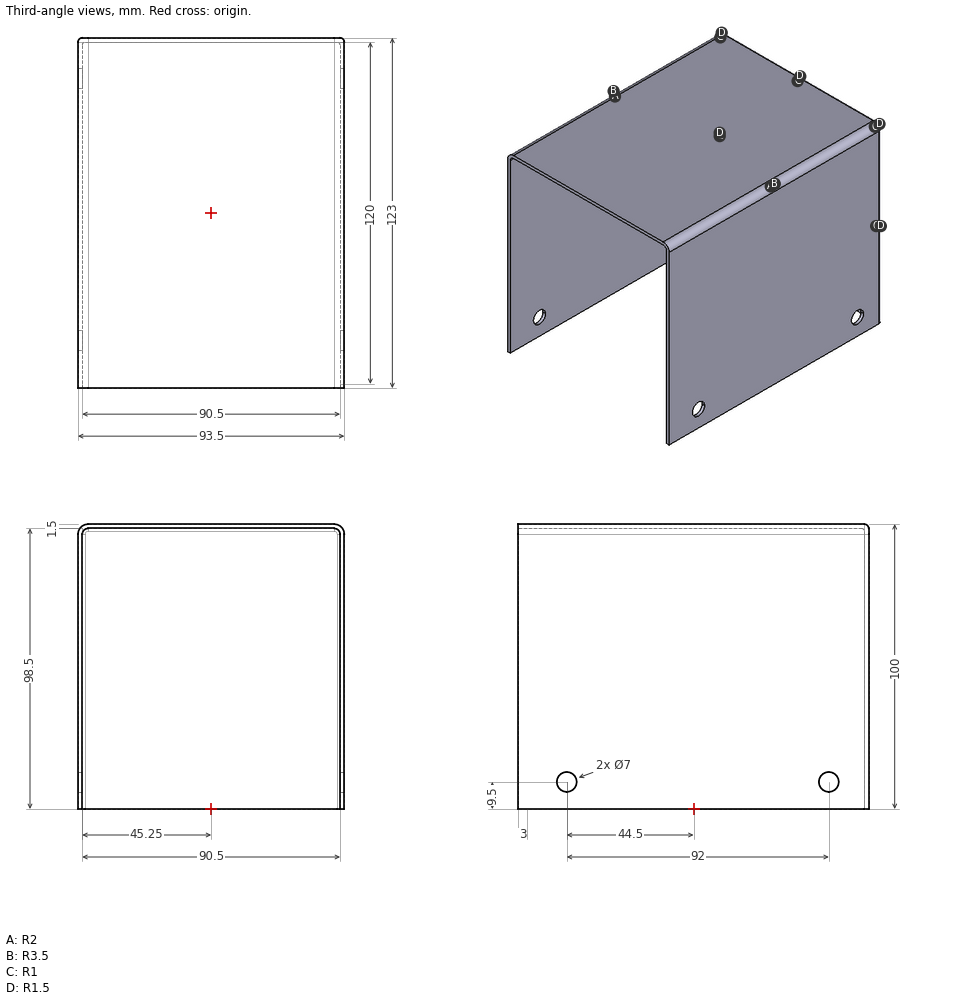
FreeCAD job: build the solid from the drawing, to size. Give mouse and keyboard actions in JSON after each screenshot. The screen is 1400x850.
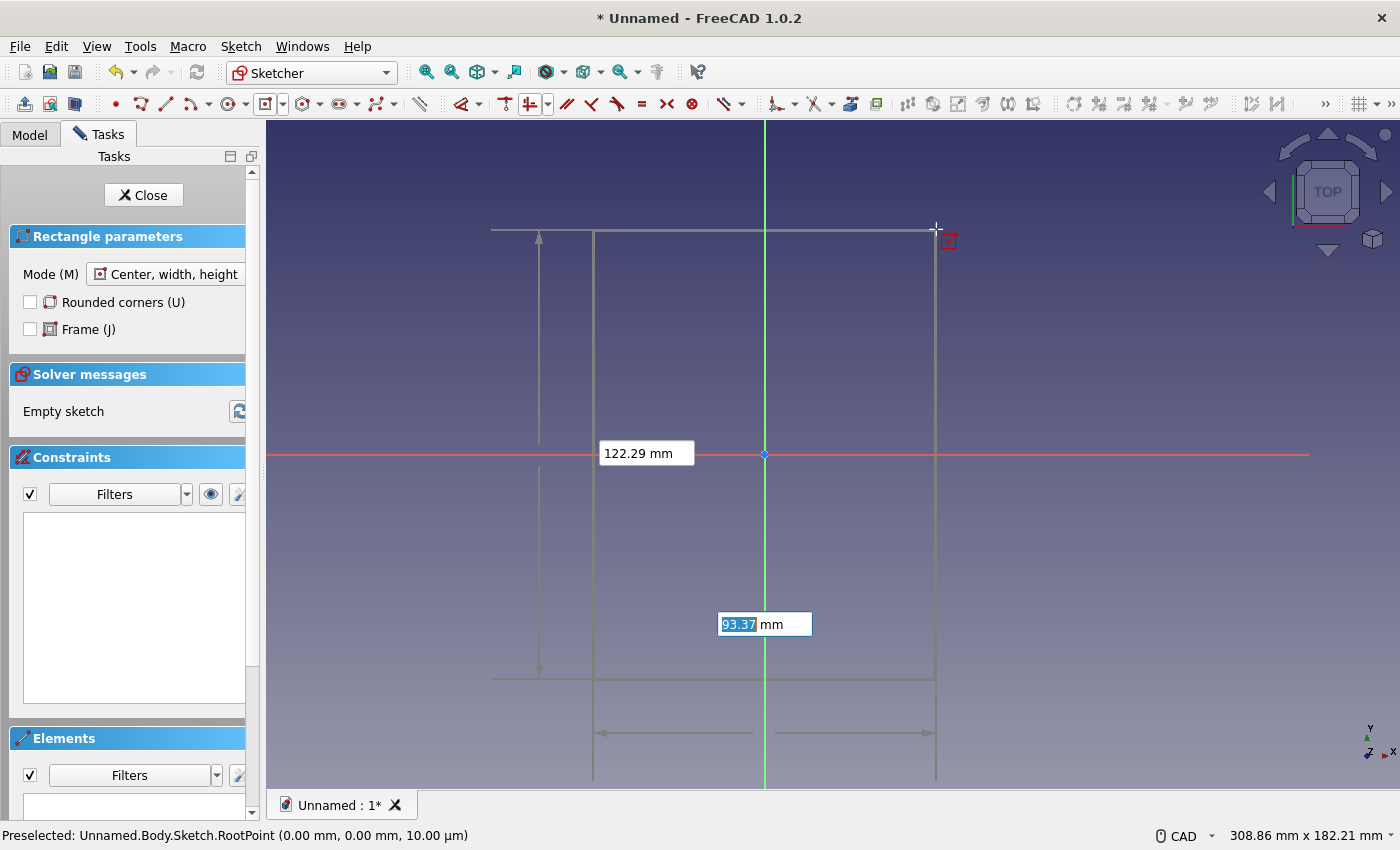
{"action": "type", "text": "93.5"}
{"action": "key", "text": "Tab"}
{"action": "type", "text": "123"}
{"action": "key", "text": "Return"}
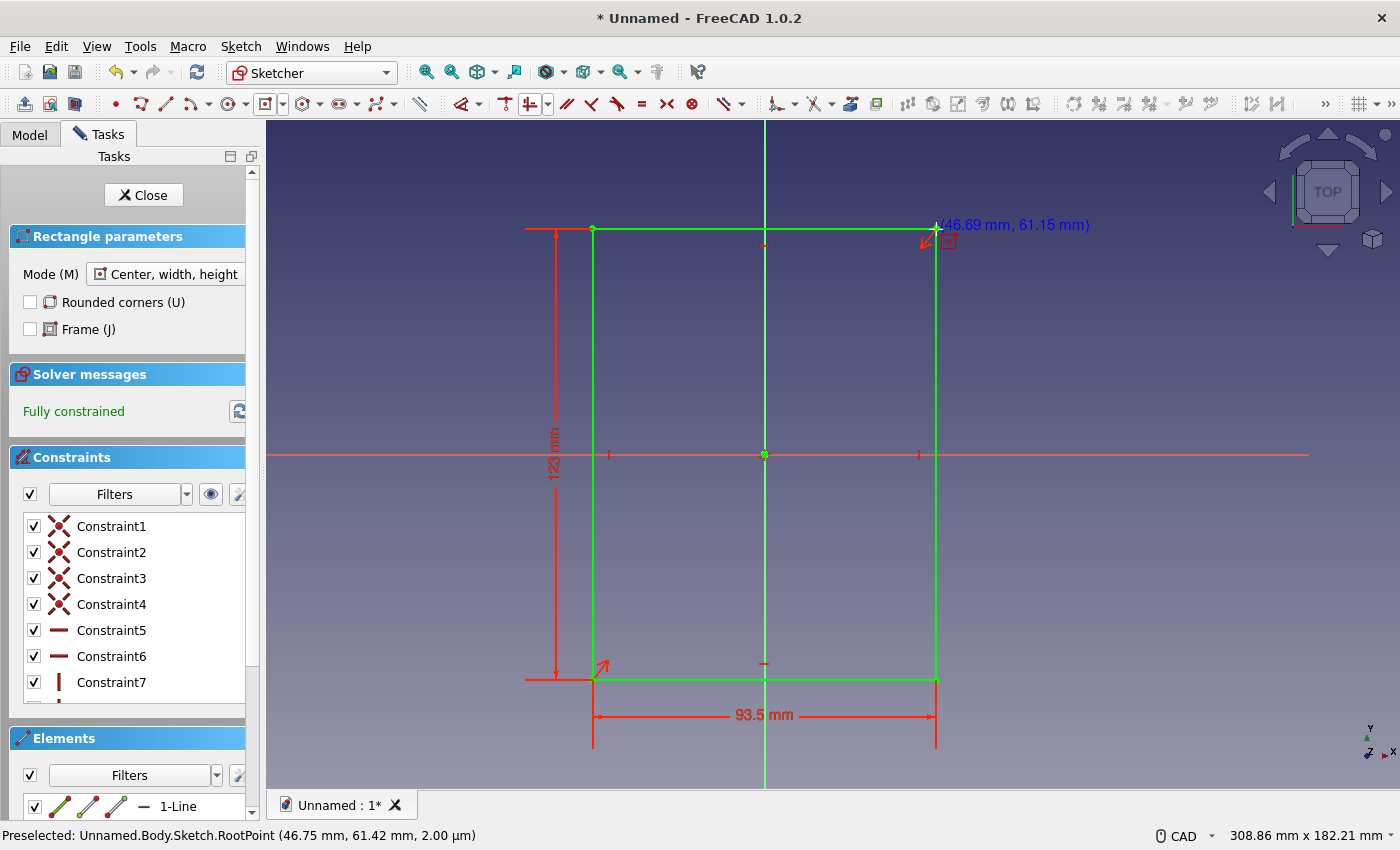
{"action": "left_click", "coordinate": [765, 454]}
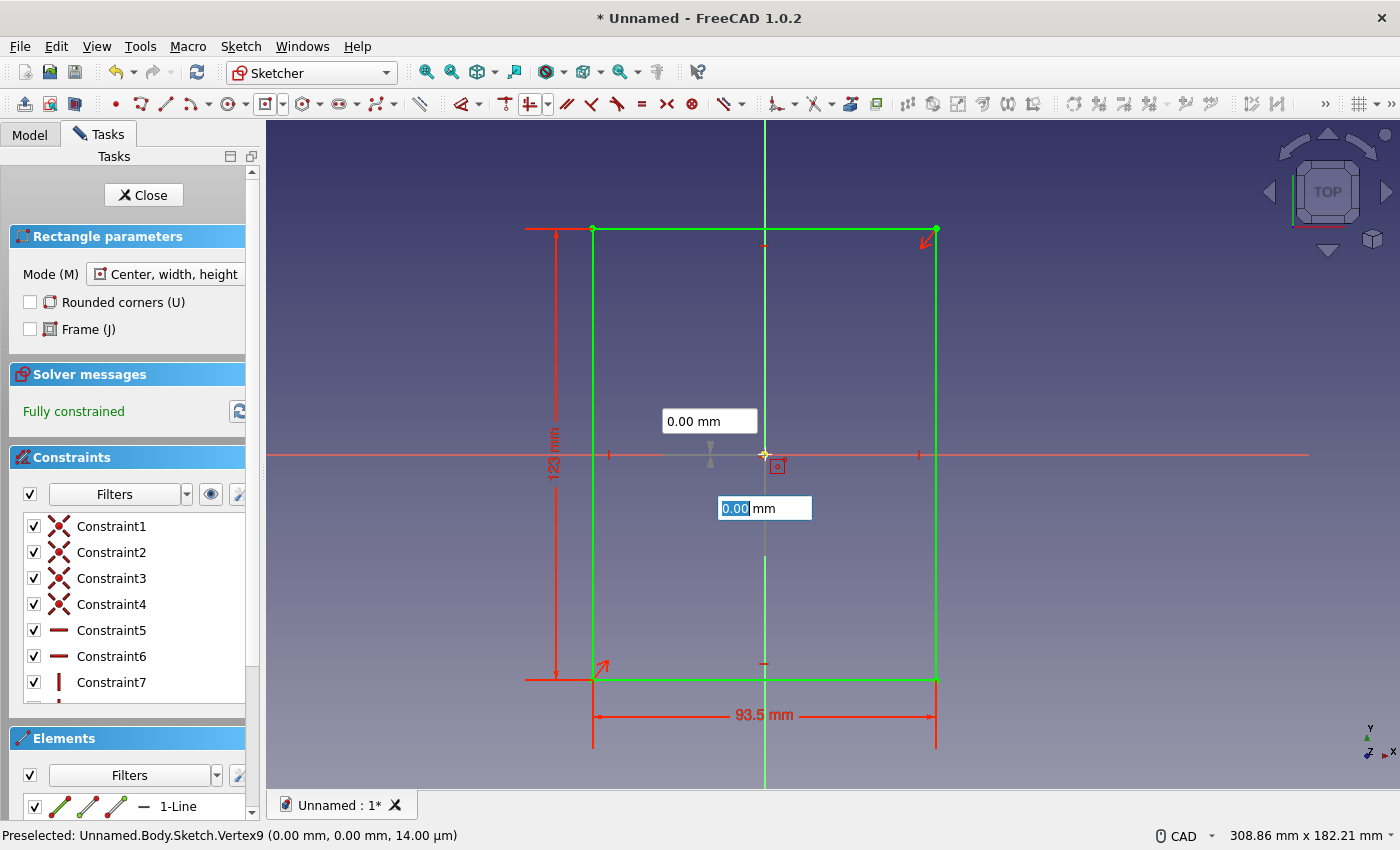
{"action": "scroll", "coordinate": [931, 234], "scroll_direction": "up", "scroll_amount": 6}
{"action": "mouse_move", "coordinate": [929, 234]}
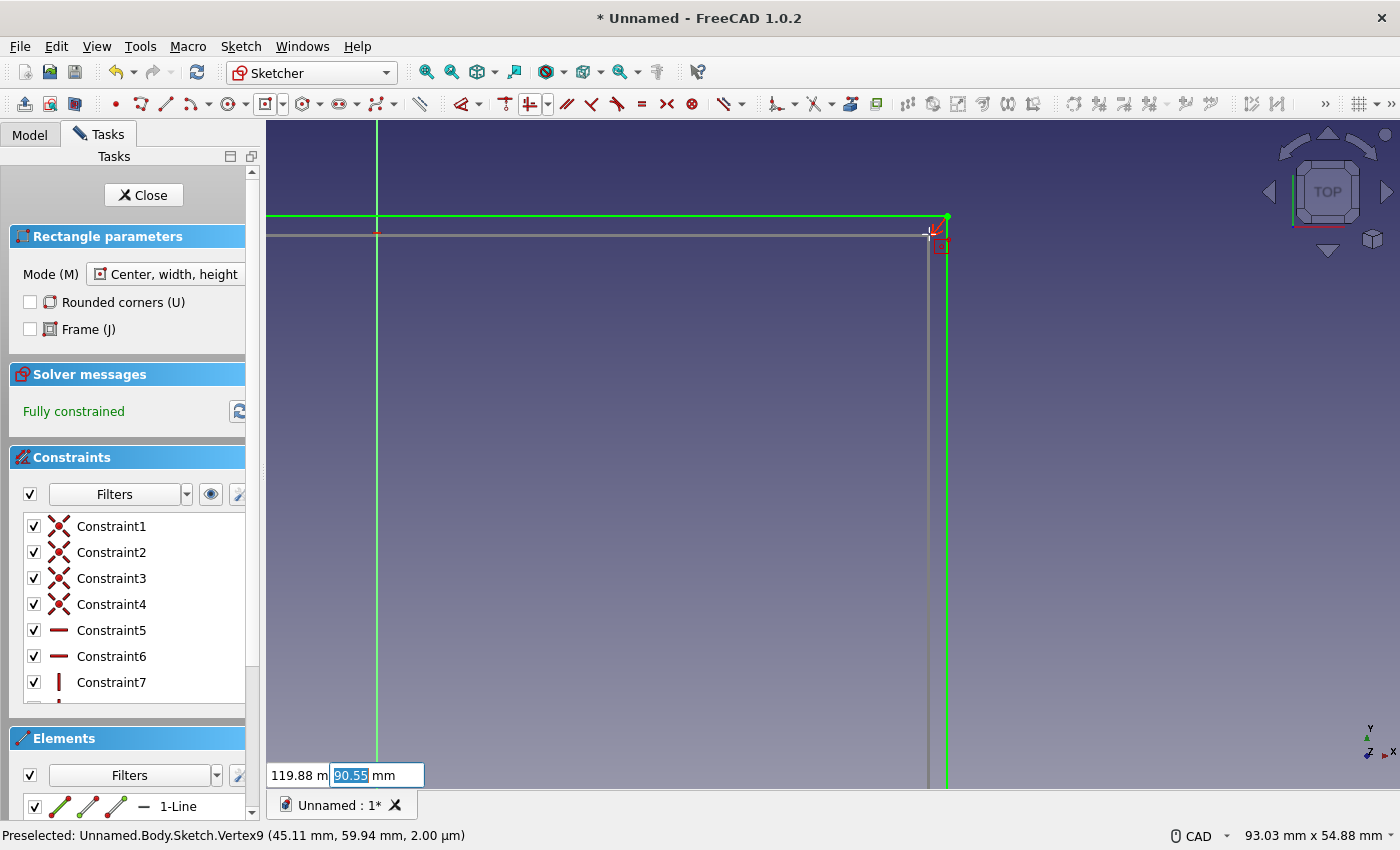
{"action": "type", "text": "90.5"}
{"action": "key", "text": "Tab"}
{"action": "type", "text": "120"}
{"action": "key", "text": "Return"}
{"action": "key", "text": "Escape"}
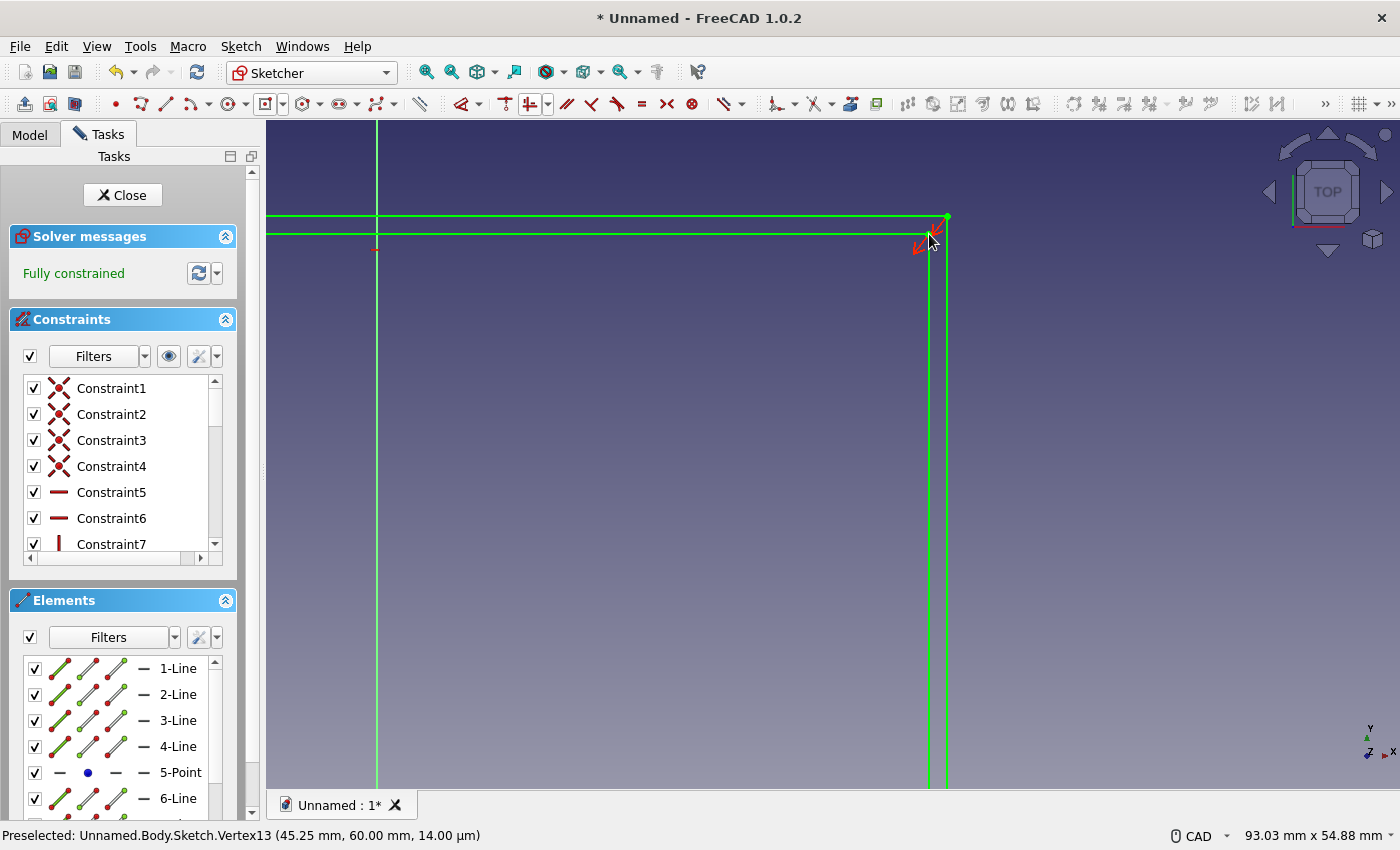
{"action": "left_click", "coordinate": [123, 195]}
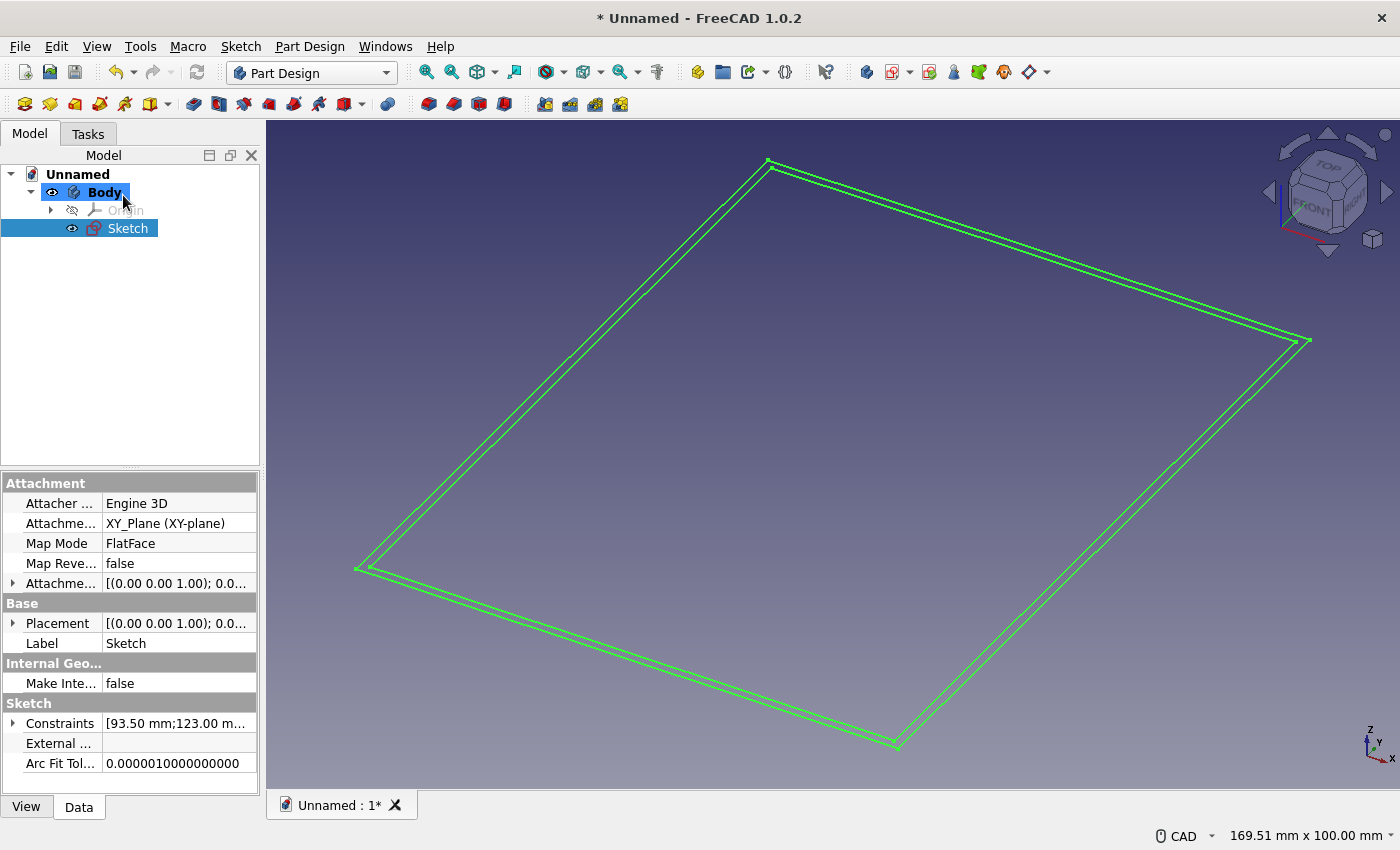
{"action": "left_click", "coordinate": [25, 104]}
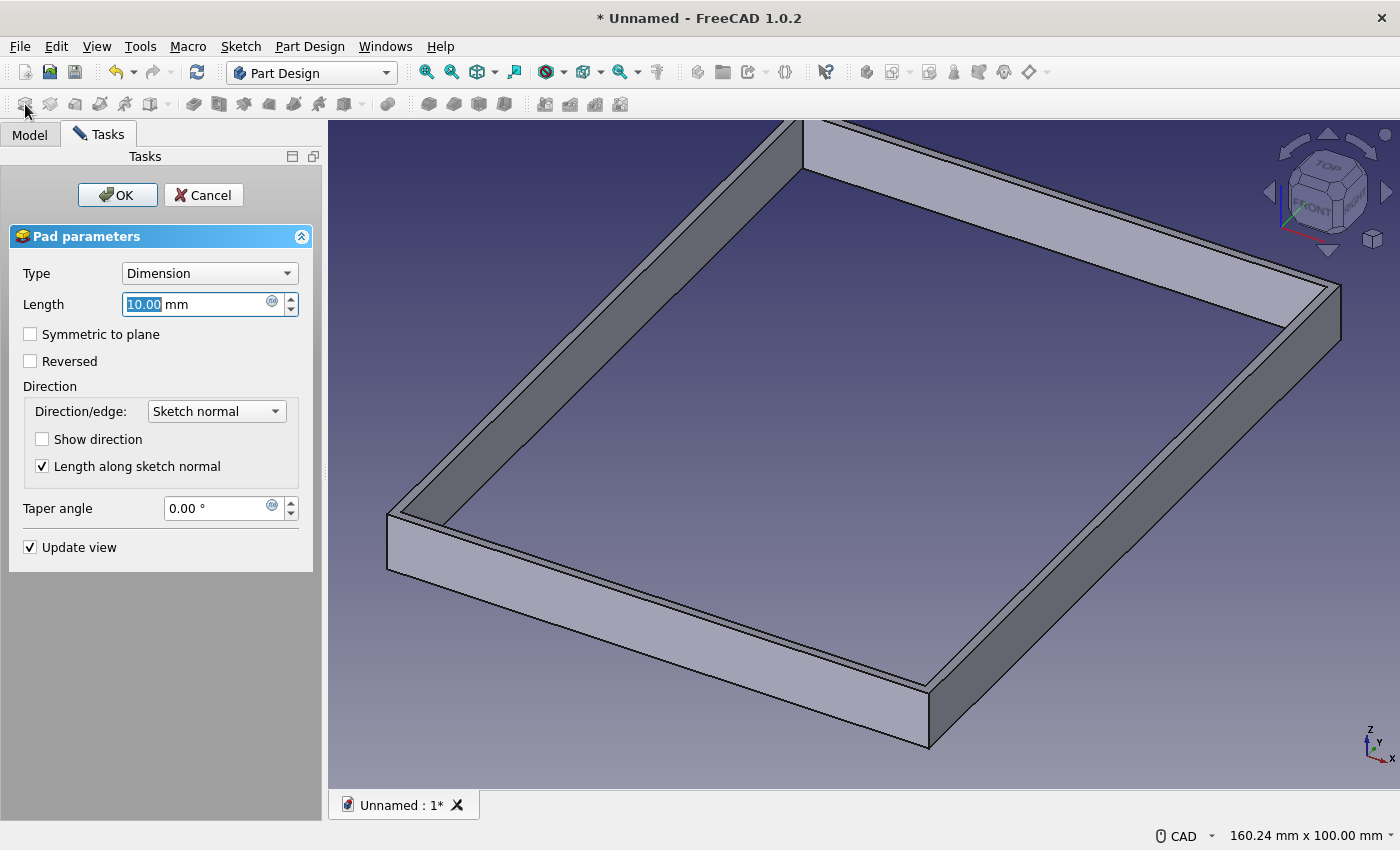
{"action": "type", "text": "100"}
{"action": "key", "text": "Tab"}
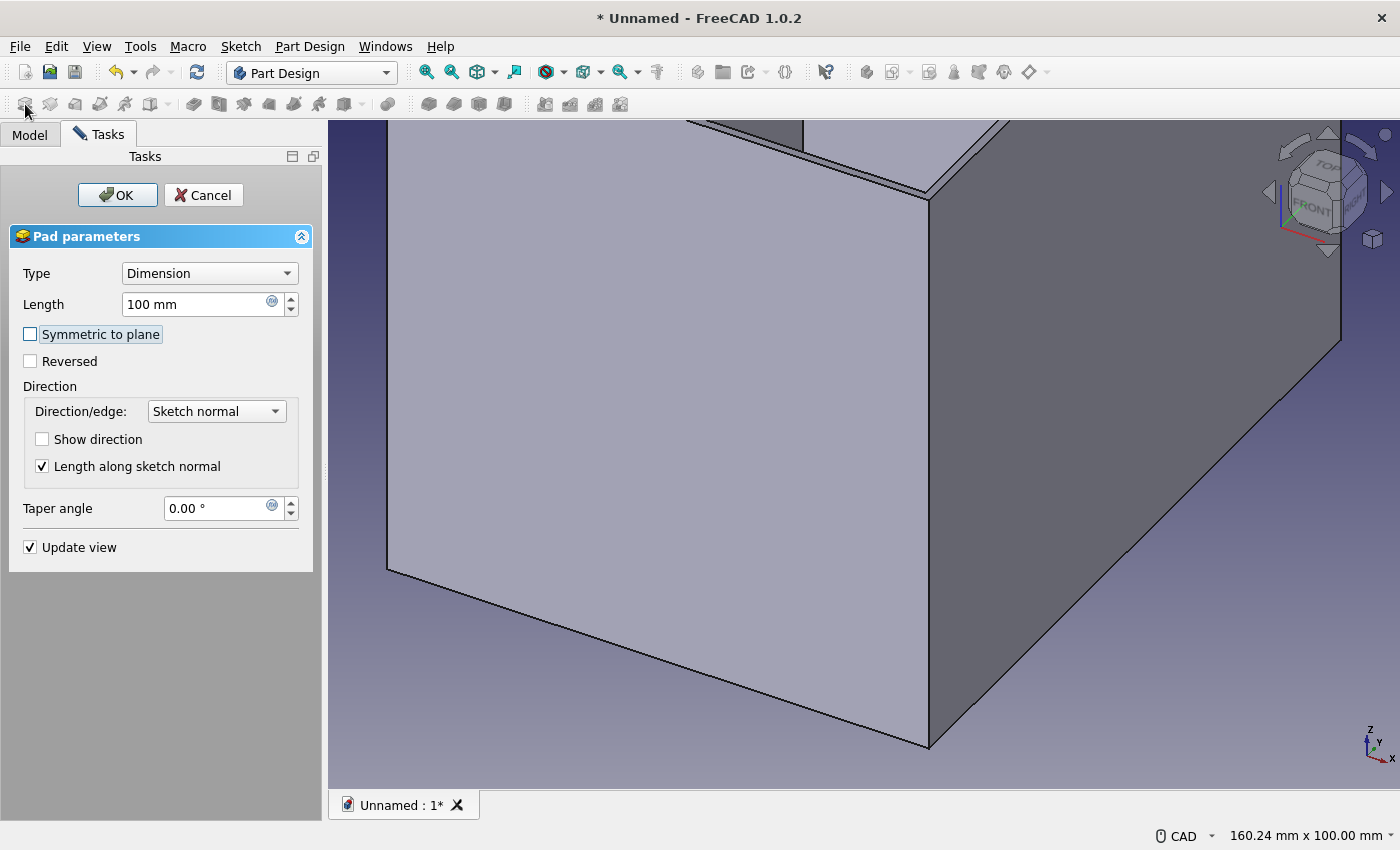
{"action": "left_click", "coordinate": [118, 195]}